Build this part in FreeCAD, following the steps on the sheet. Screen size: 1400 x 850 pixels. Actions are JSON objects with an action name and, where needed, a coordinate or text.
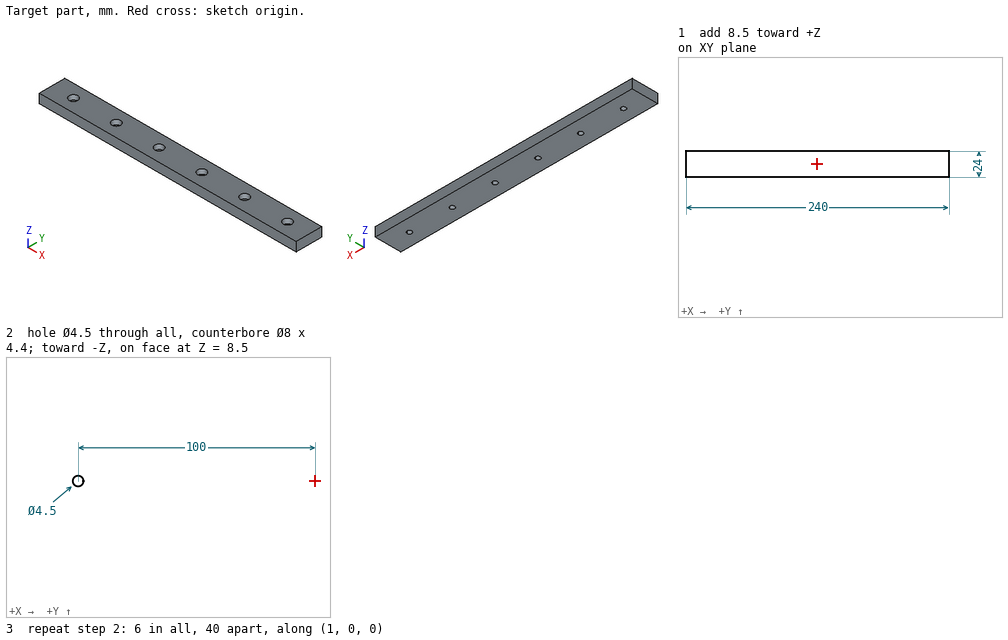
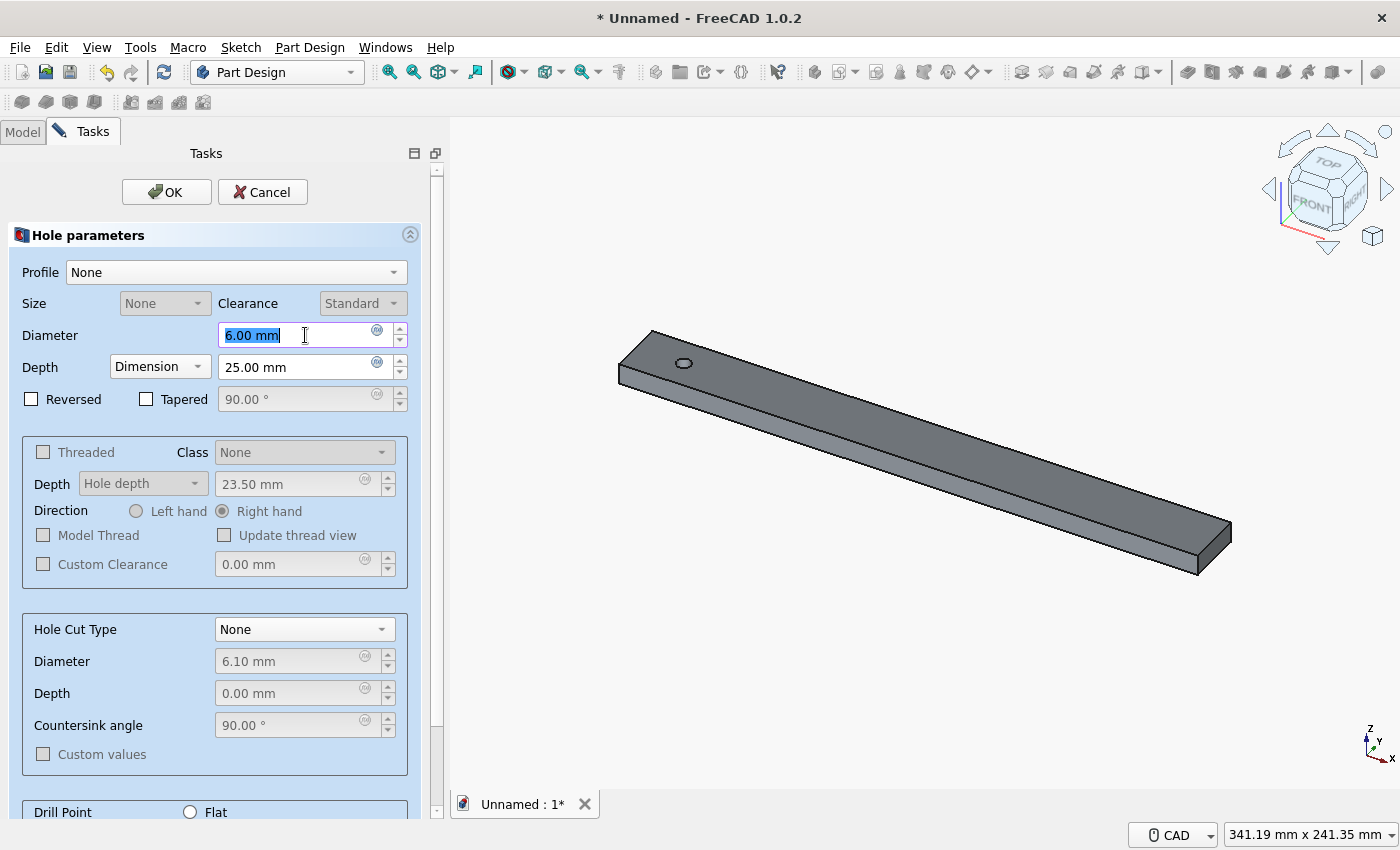
{"action": "type", "text": "4.5"}
{"action": "key", "text": "Tab"}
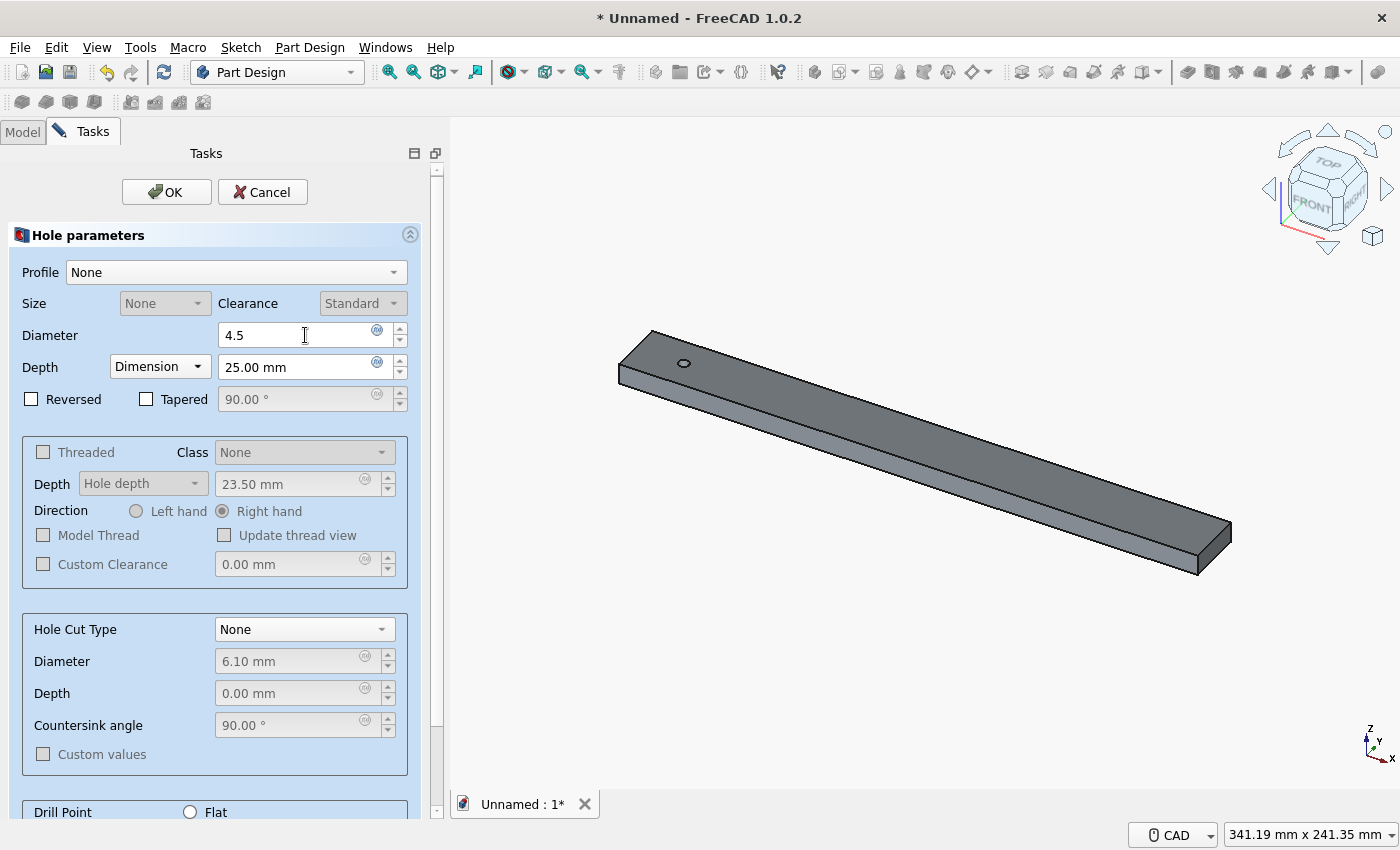
{"action": "left_click", "coordinate": [161, 366]}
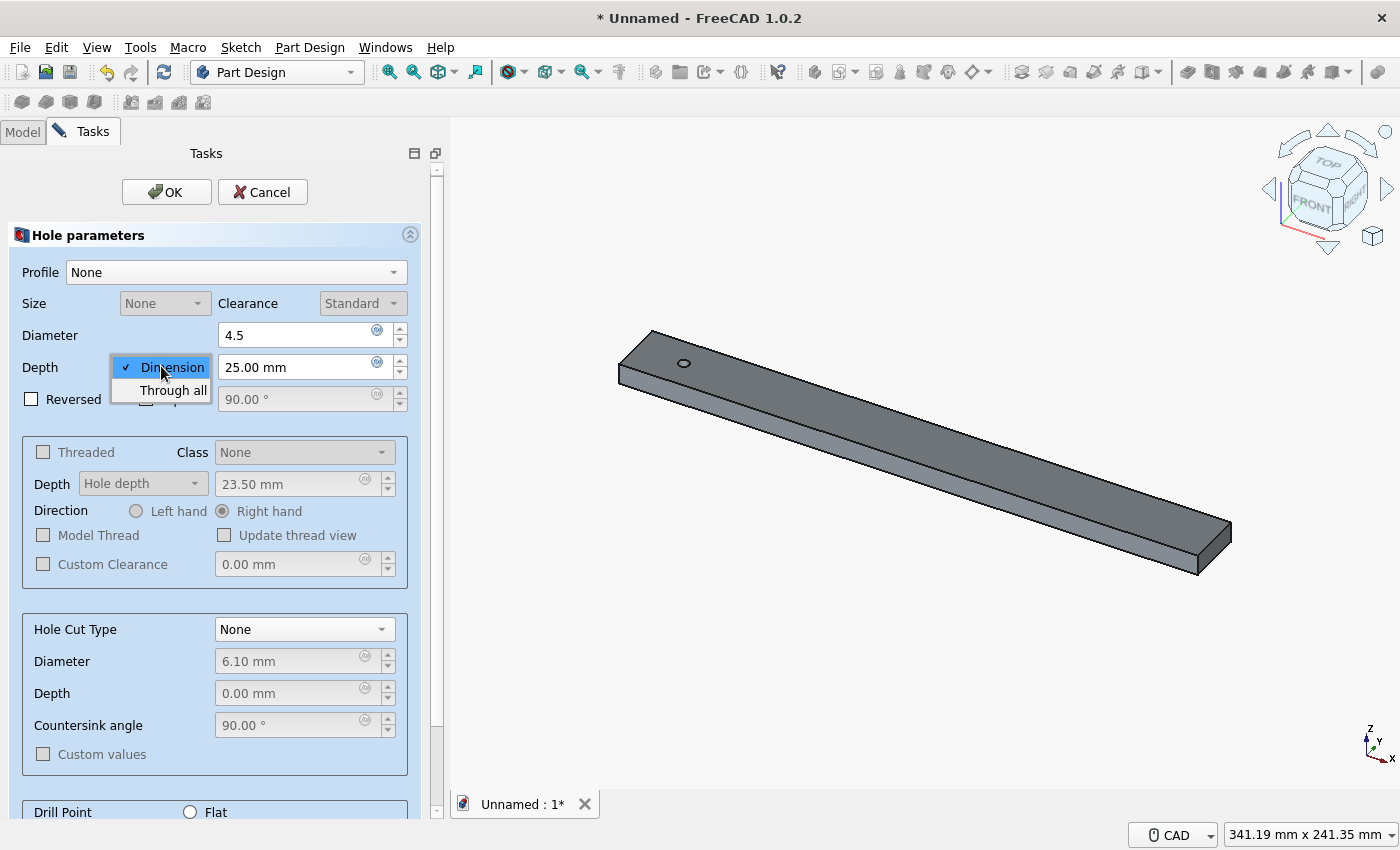
{"action": "left_click", "coordinate": [160, 390]}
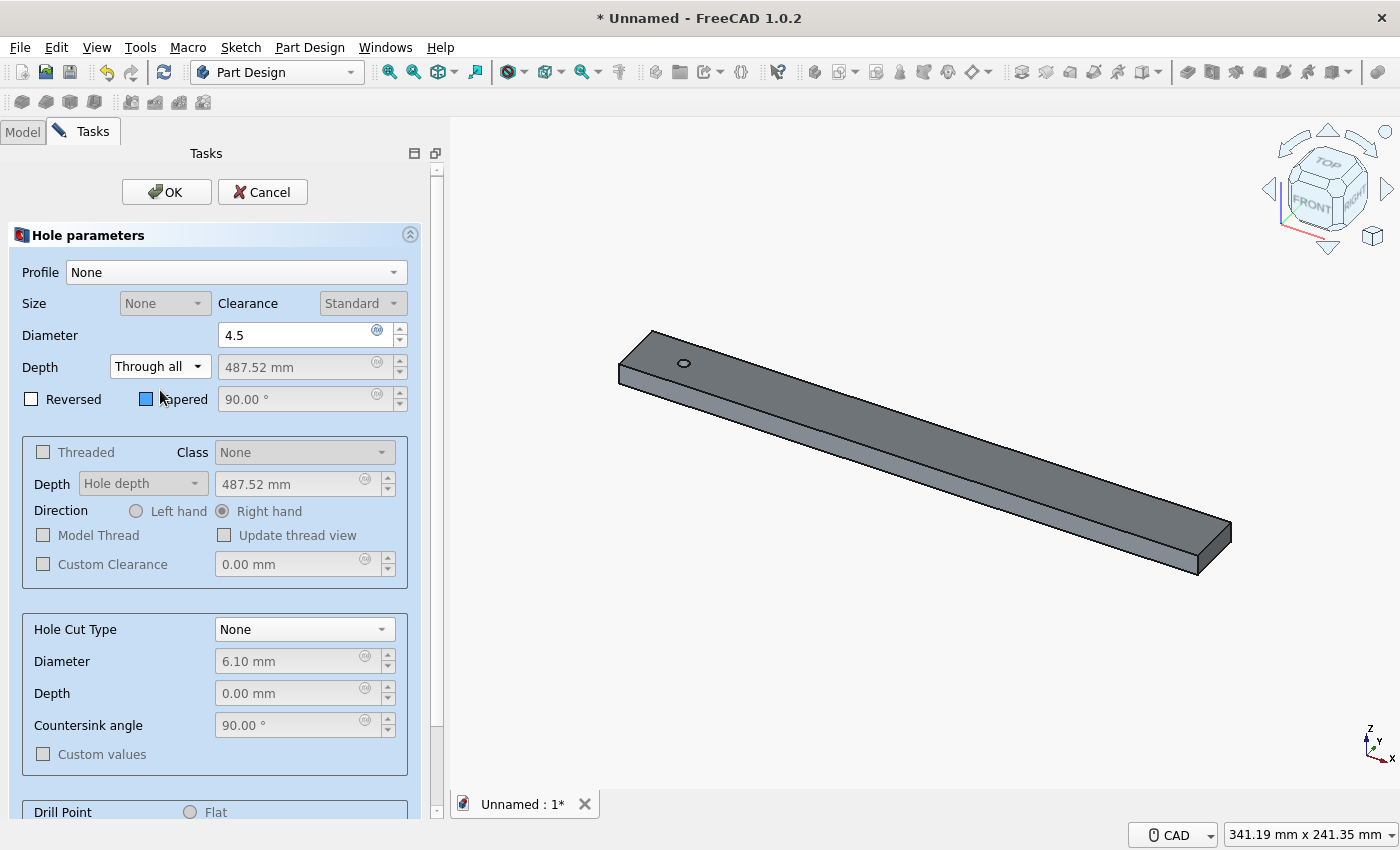
{"action": "left_click", "coordinate": [306, 630]}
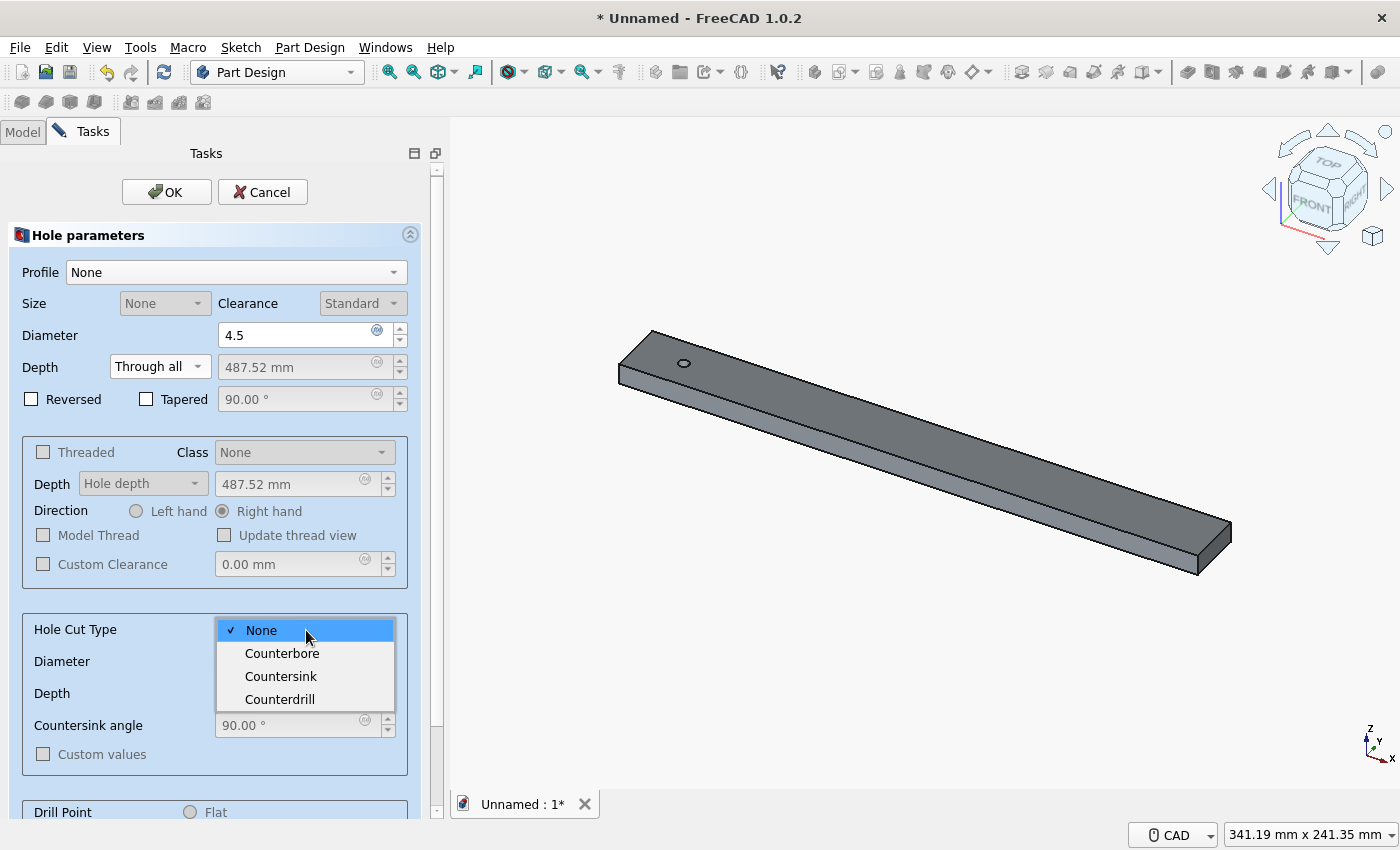
{"action": "left_click", "coordinate": [304, 654]}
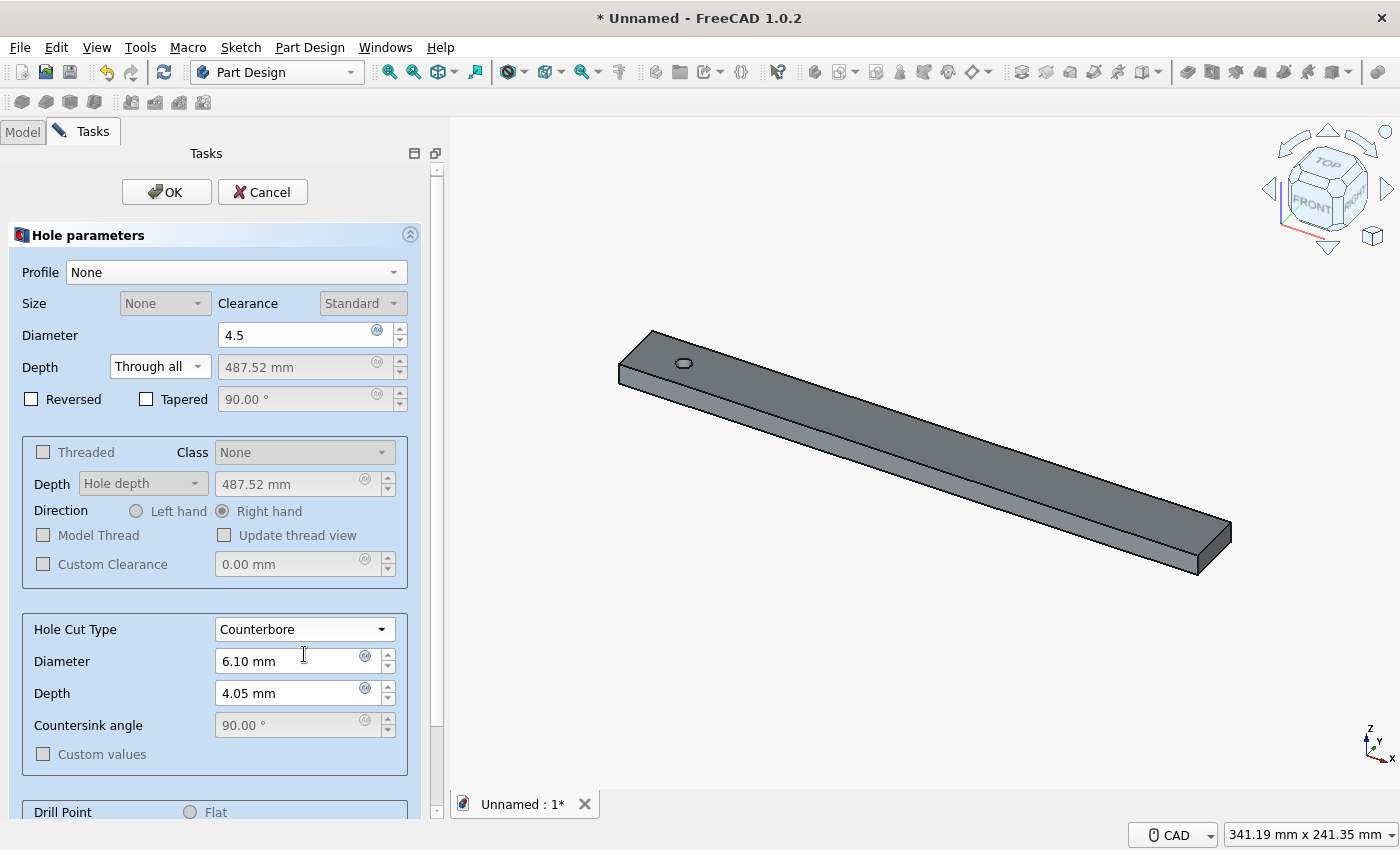
{"action": "triple_click", "coordinate": [298, 661]}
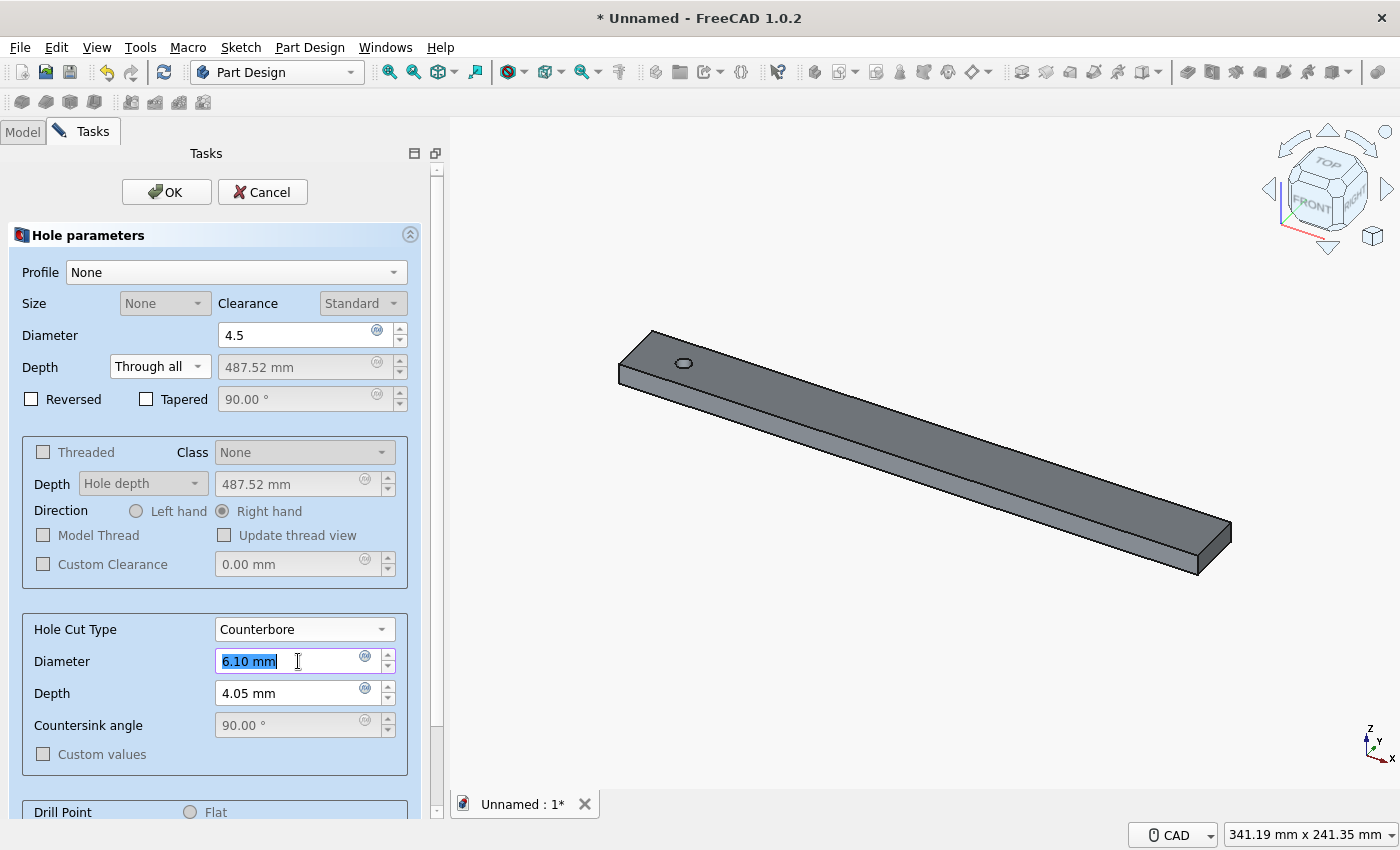
{"action": "type", "text": "8"}
{"action": "key", "text": "Tab"}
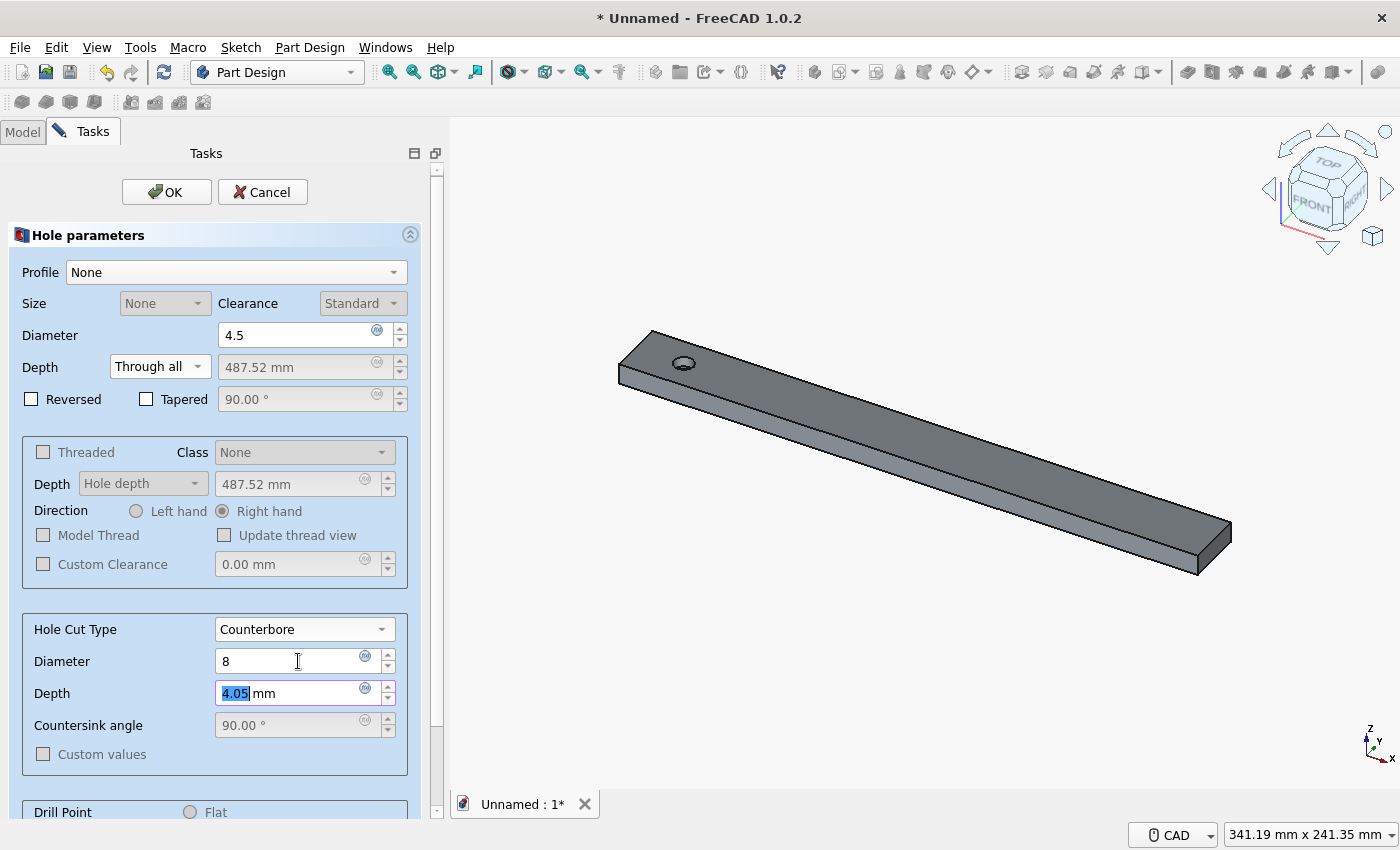
{"action": "type", "text": "4.4"}
{"action": "key", "text": "Tab"}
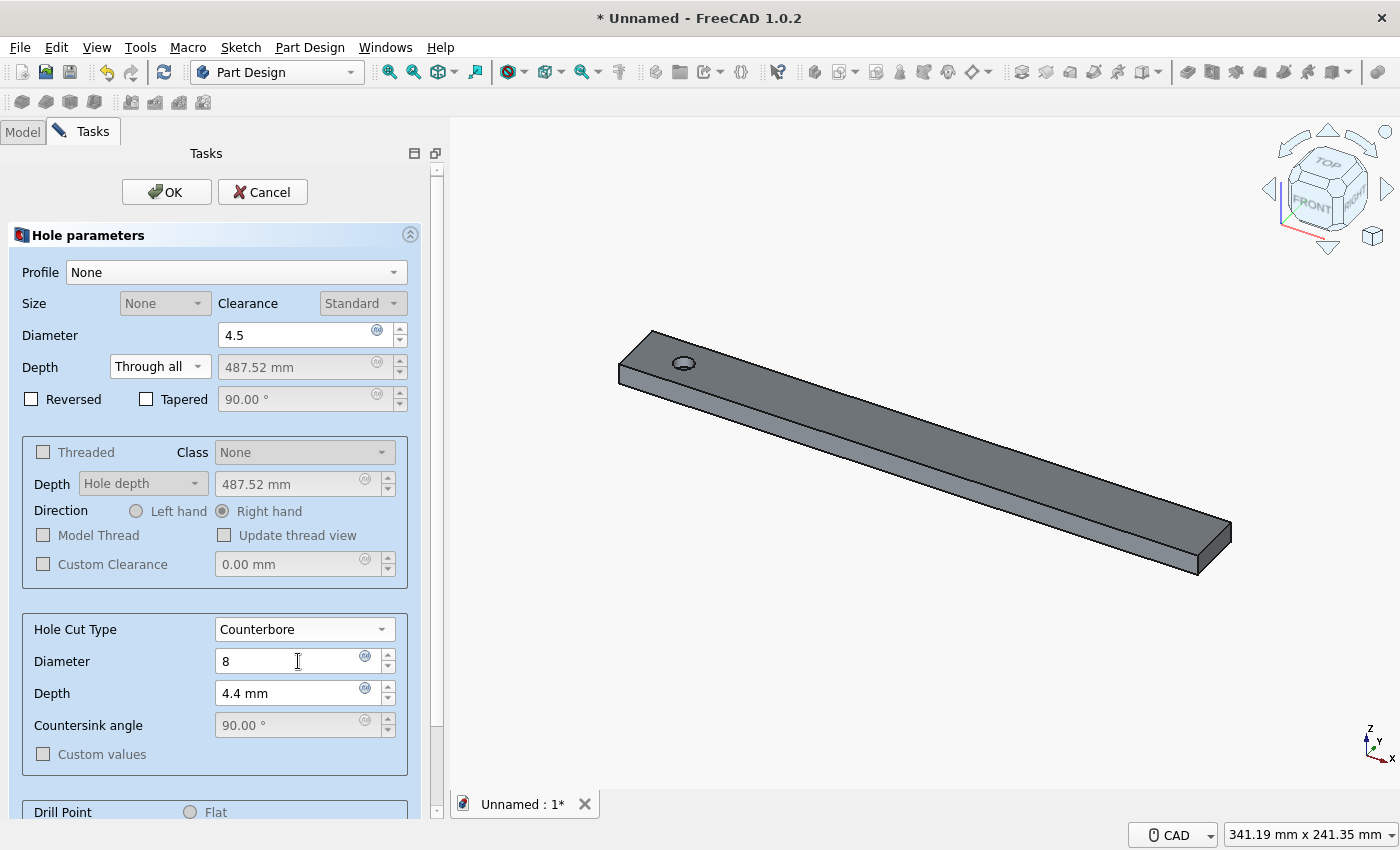
{"action": "left_click", "coordinate": [167, 192]}